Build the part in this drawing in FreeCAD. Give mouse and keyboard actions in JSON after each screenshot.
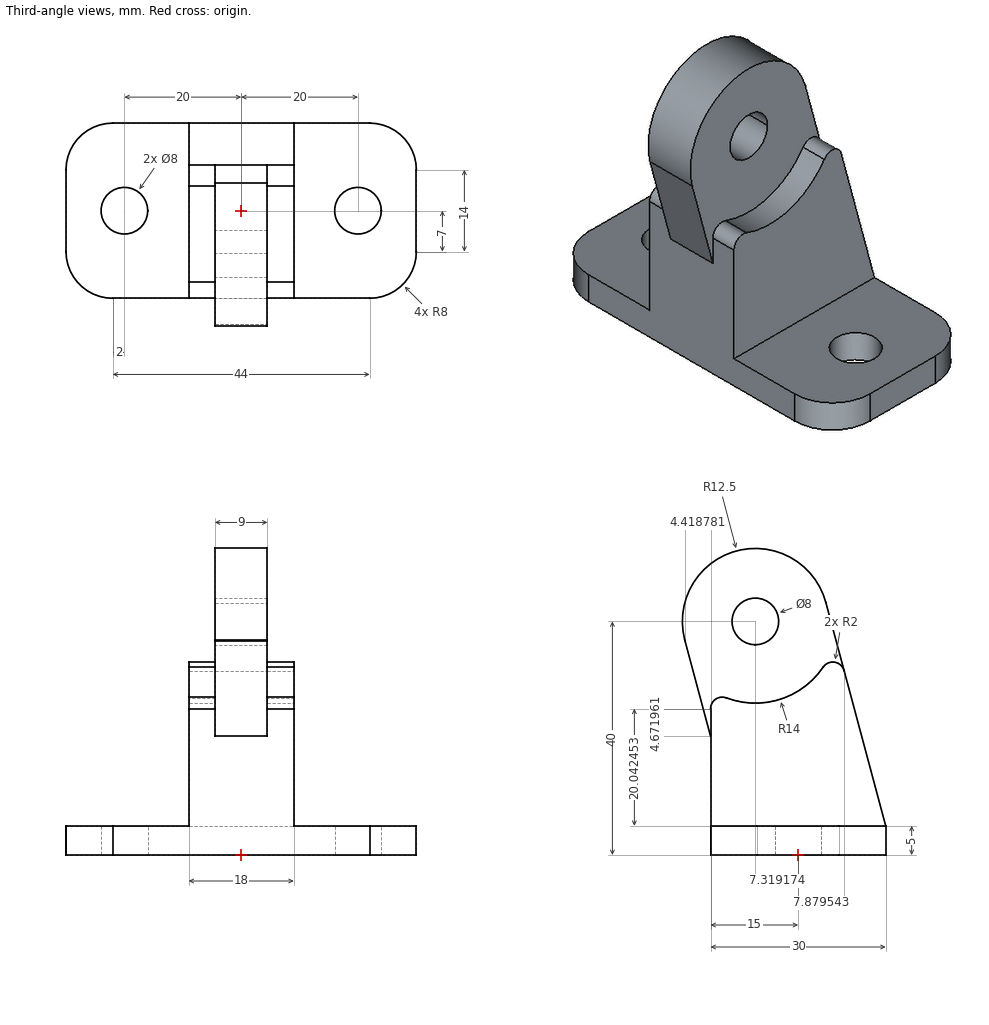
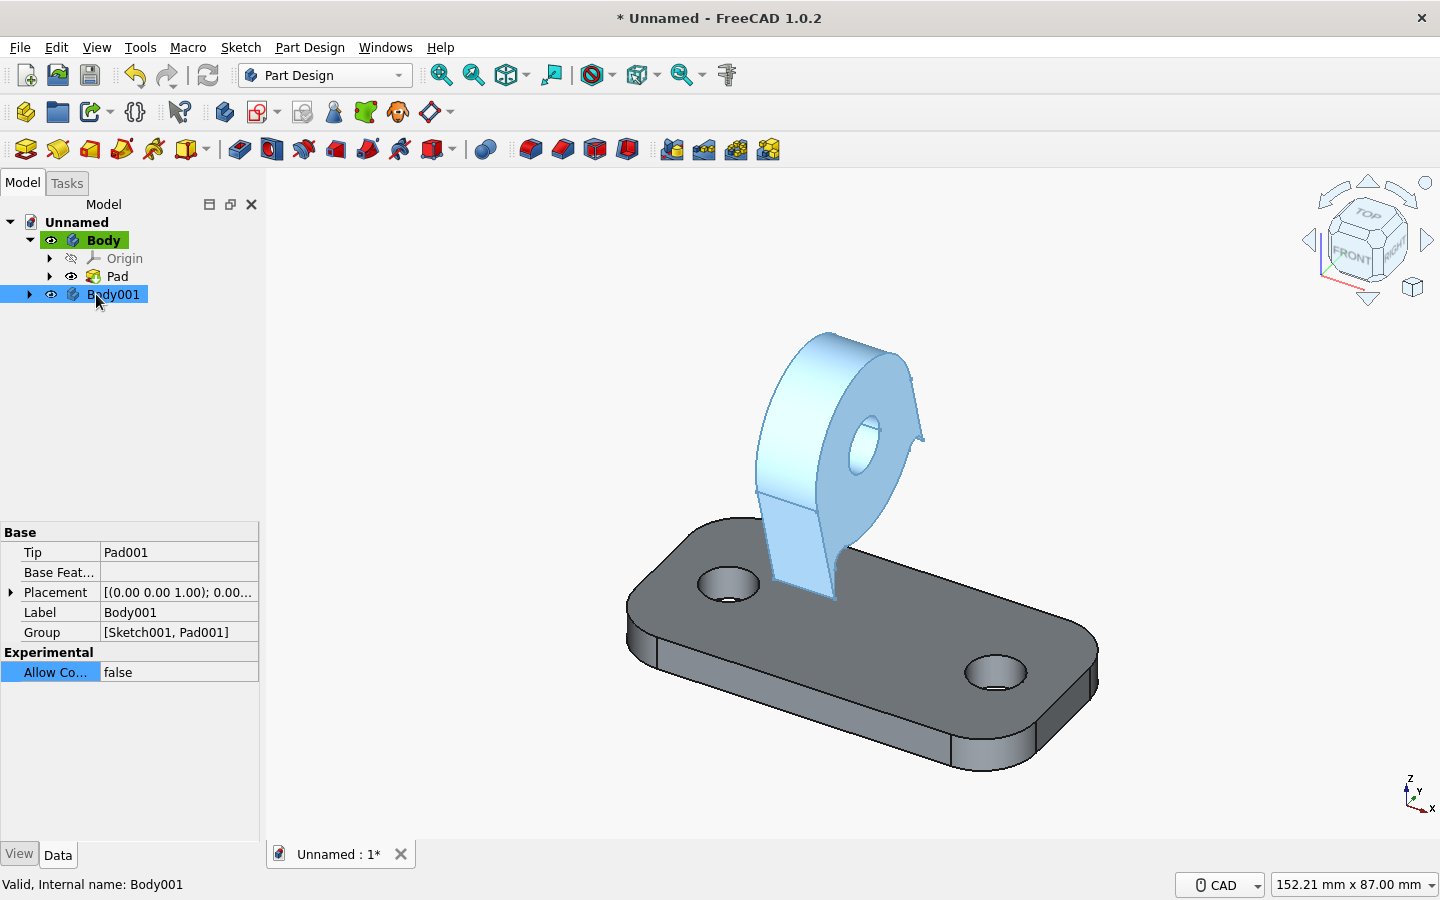
{"action": "left_click", "coordinate": [486, 150]}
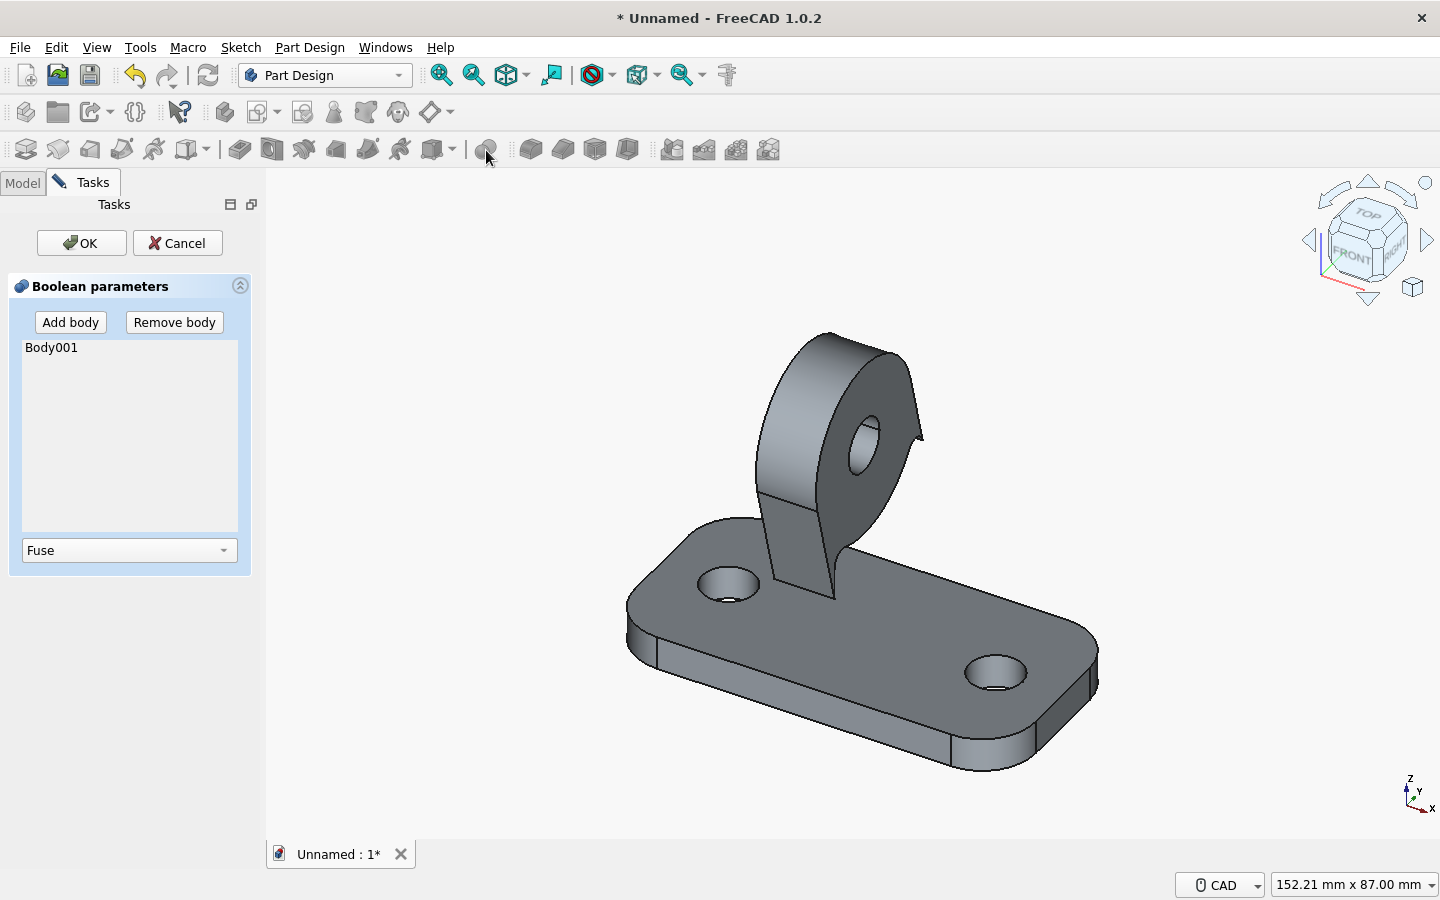
{"action": "left_click", "coordinate": [82, 243]}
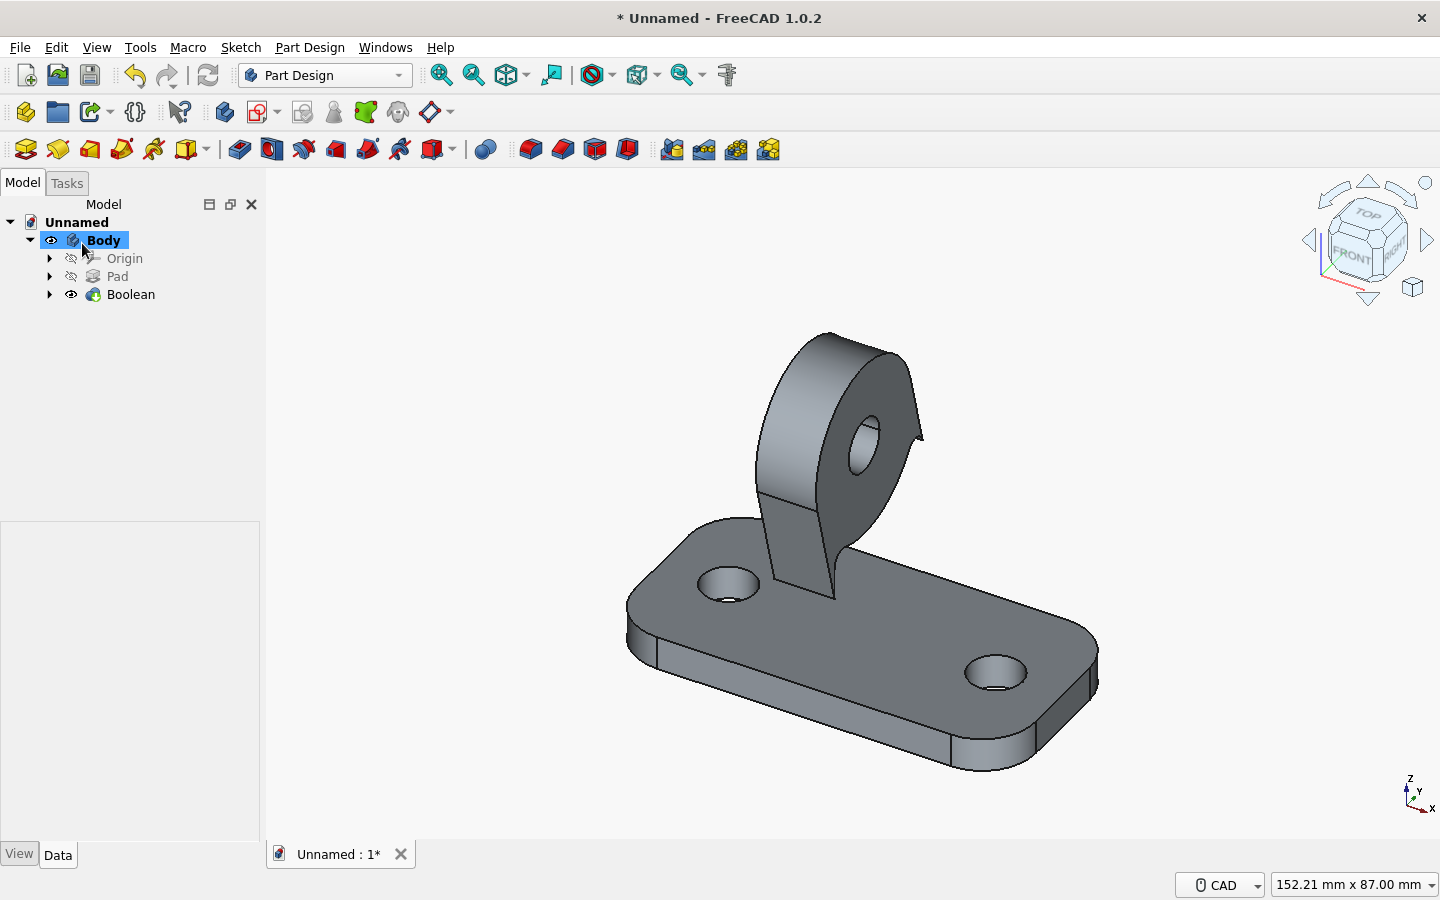
{"action": "left_click", "coordinate": [258, 112]}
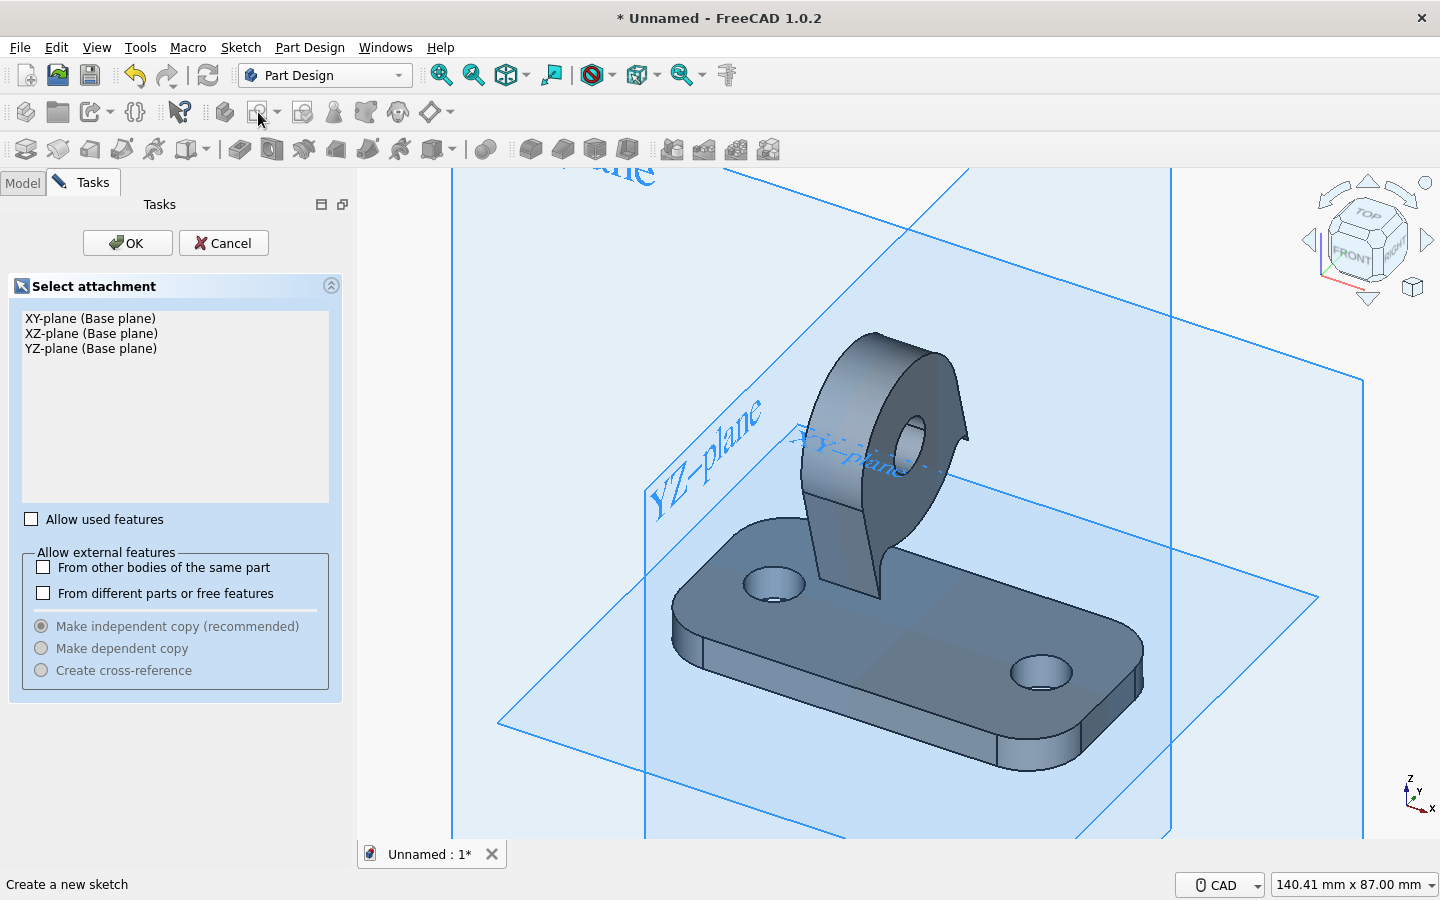
{"action": "left_click", "coordinate": [82, 348]}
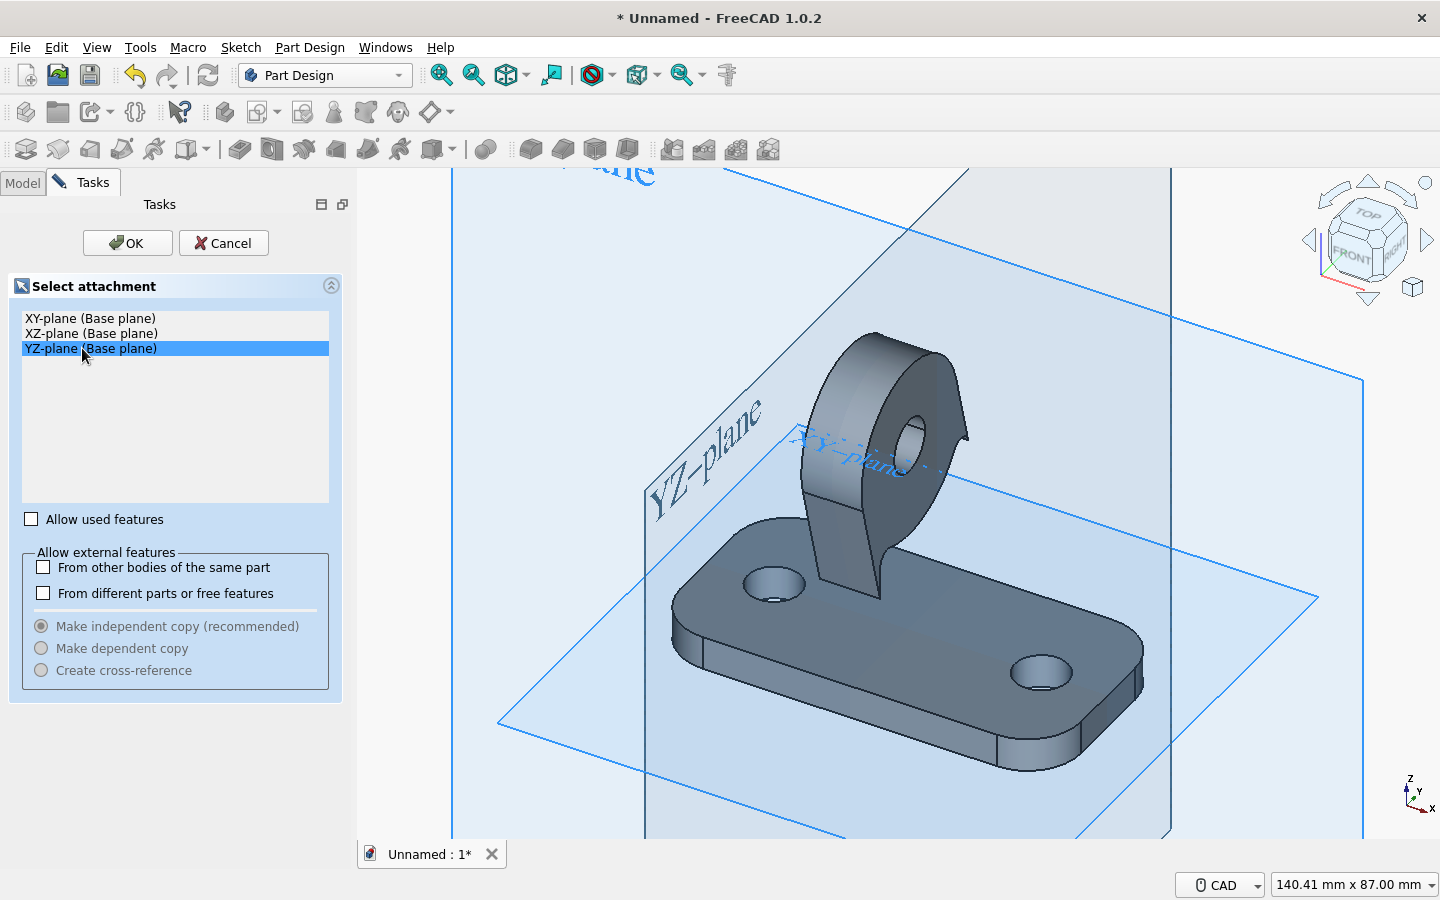
{"action": "left_click", "coordinate": [128, 243]}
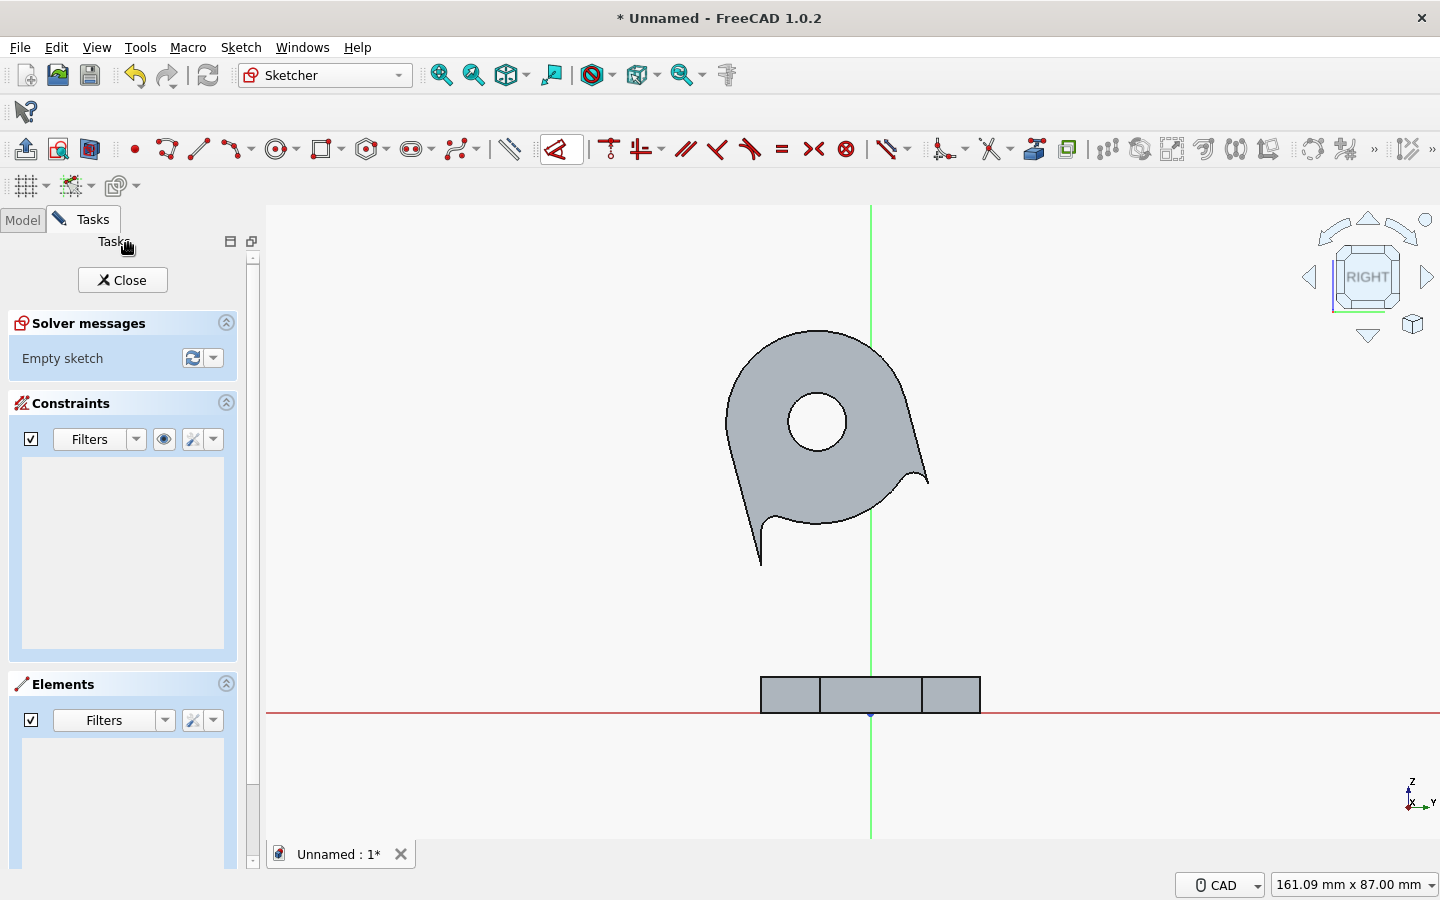
{"action": "left_click", "coordinate": [90, 150]}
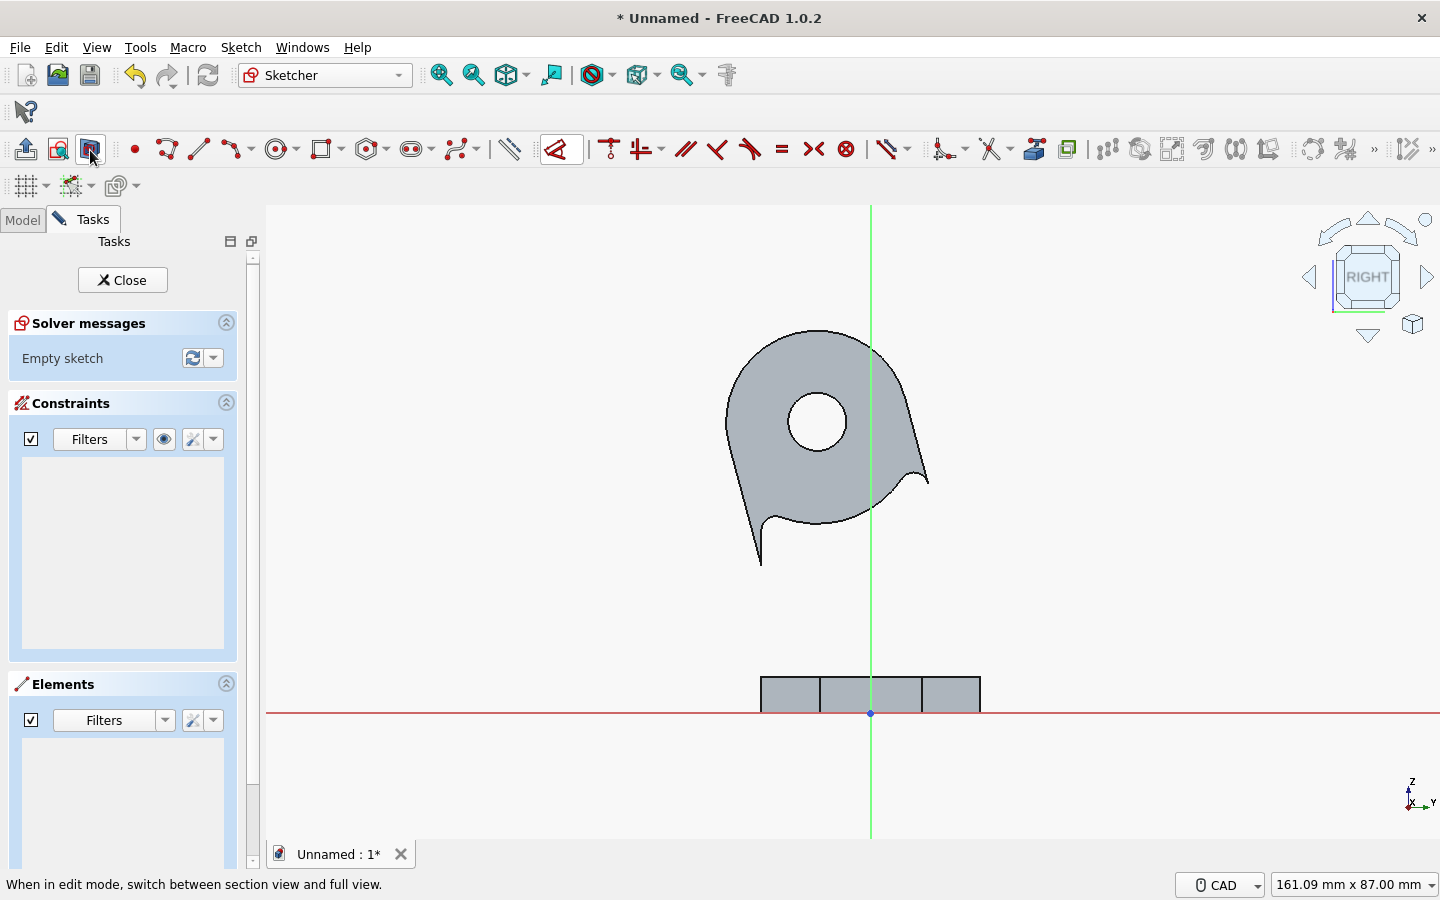
{"action": "scroll", "coordinate": [975, 679], "scroll_direction": "up", "scroll_amount": 3}